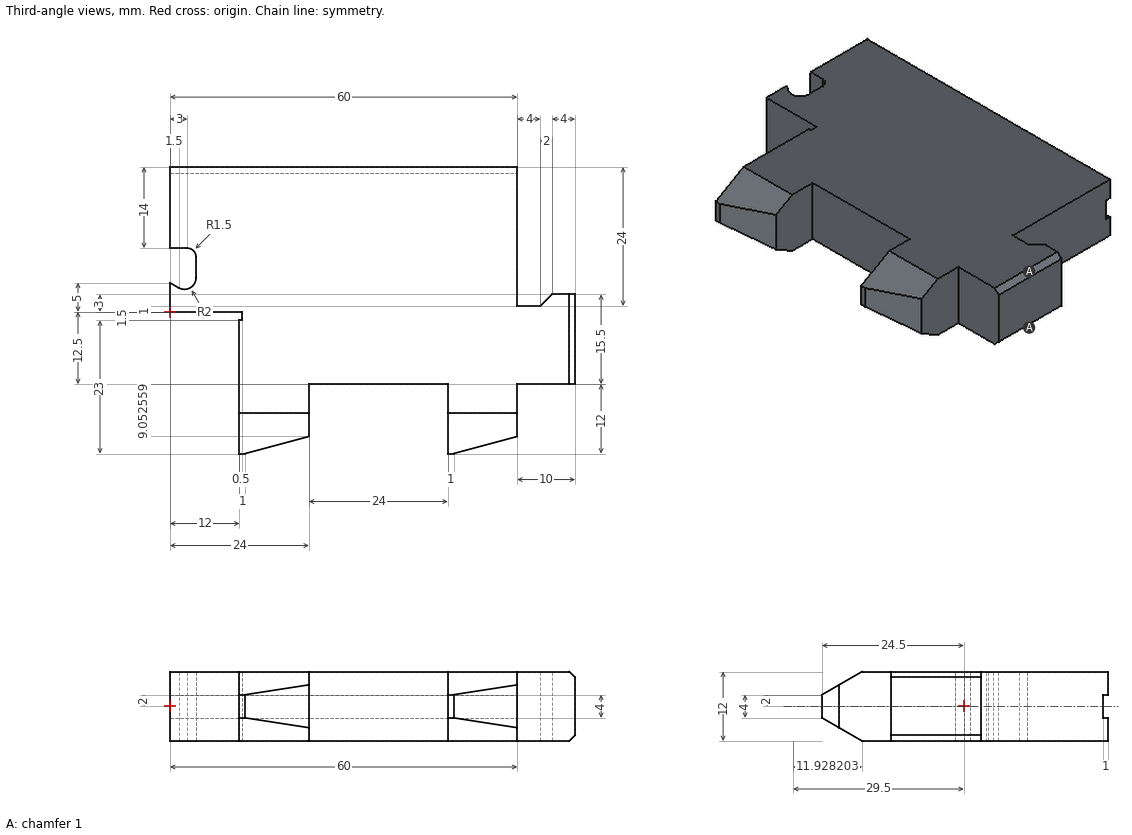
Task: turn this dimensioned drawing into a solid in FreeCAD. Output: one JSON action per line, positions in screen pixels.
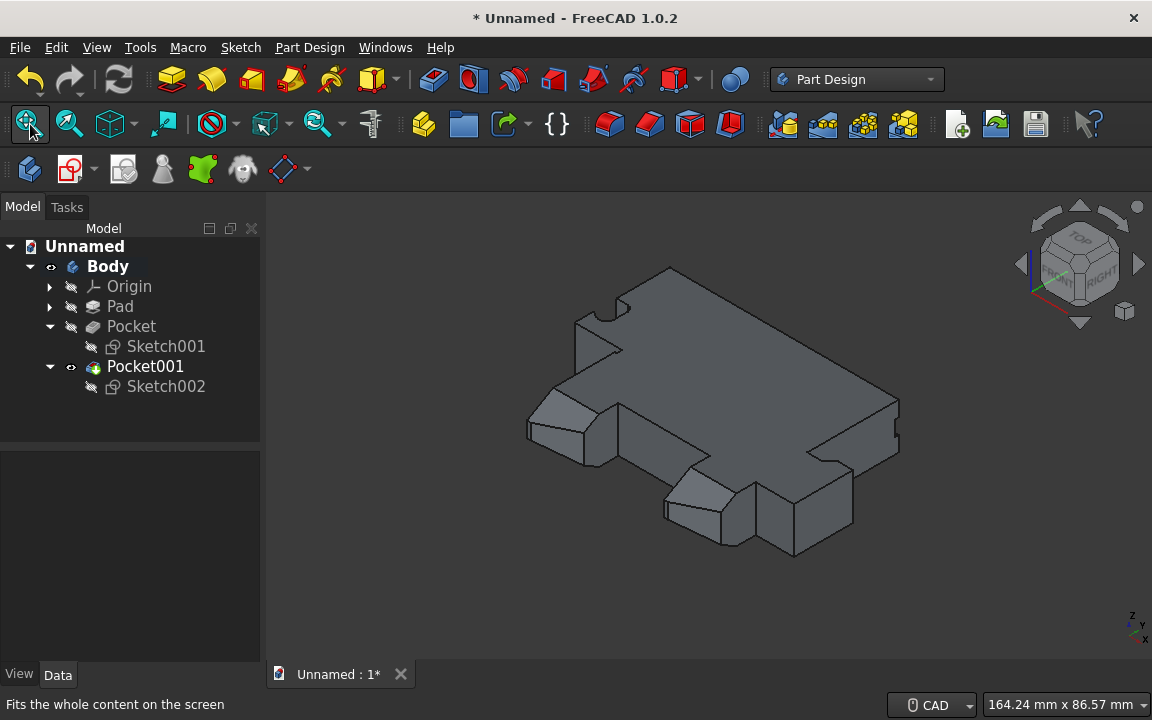
{"action": "left_click", "coordinate": [823, 486]}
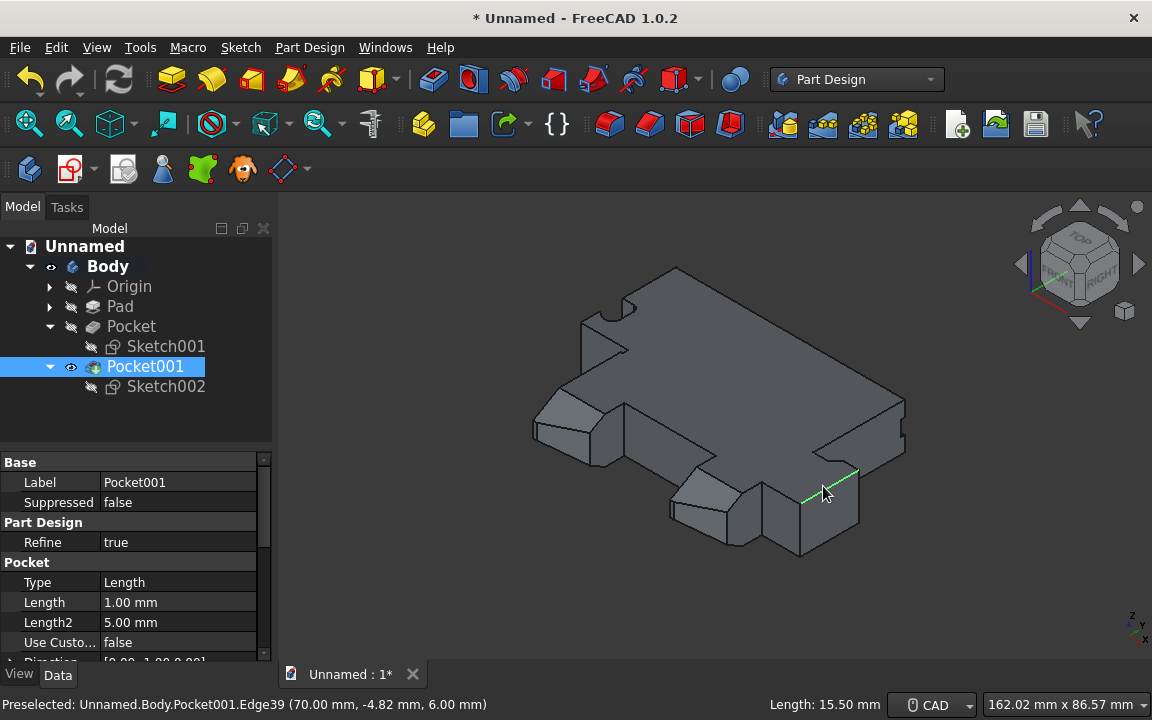
{"action": "key", "text": "2"}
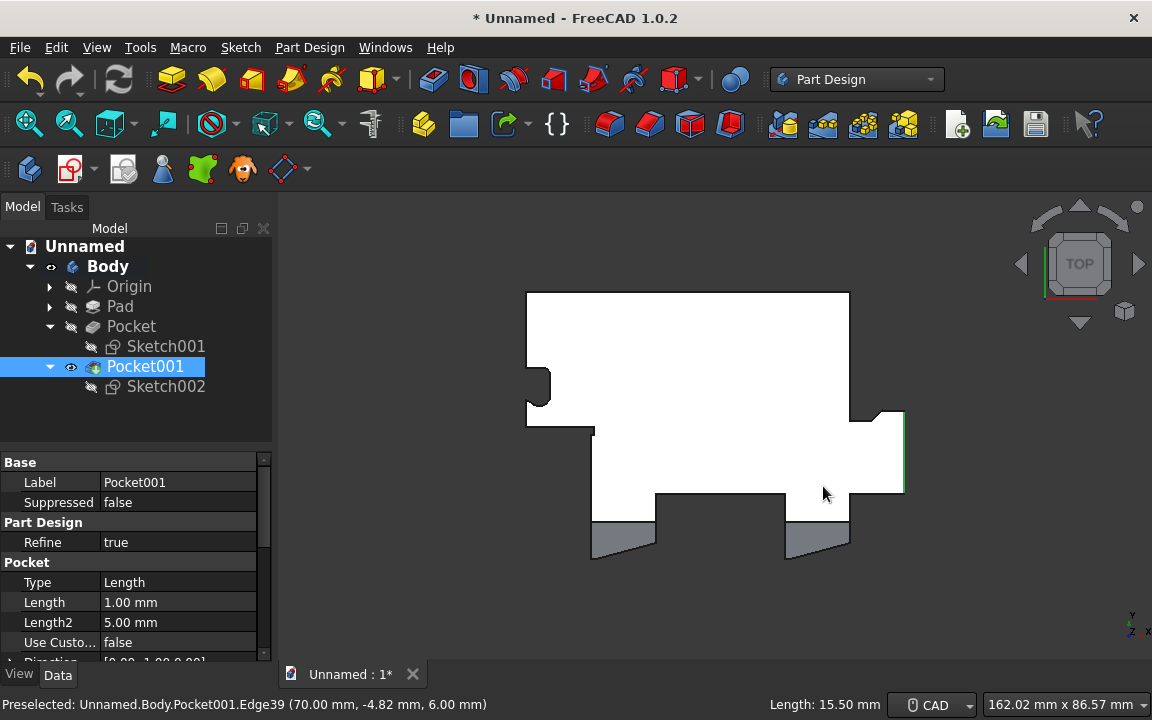
{"action": "key", "text": "1"}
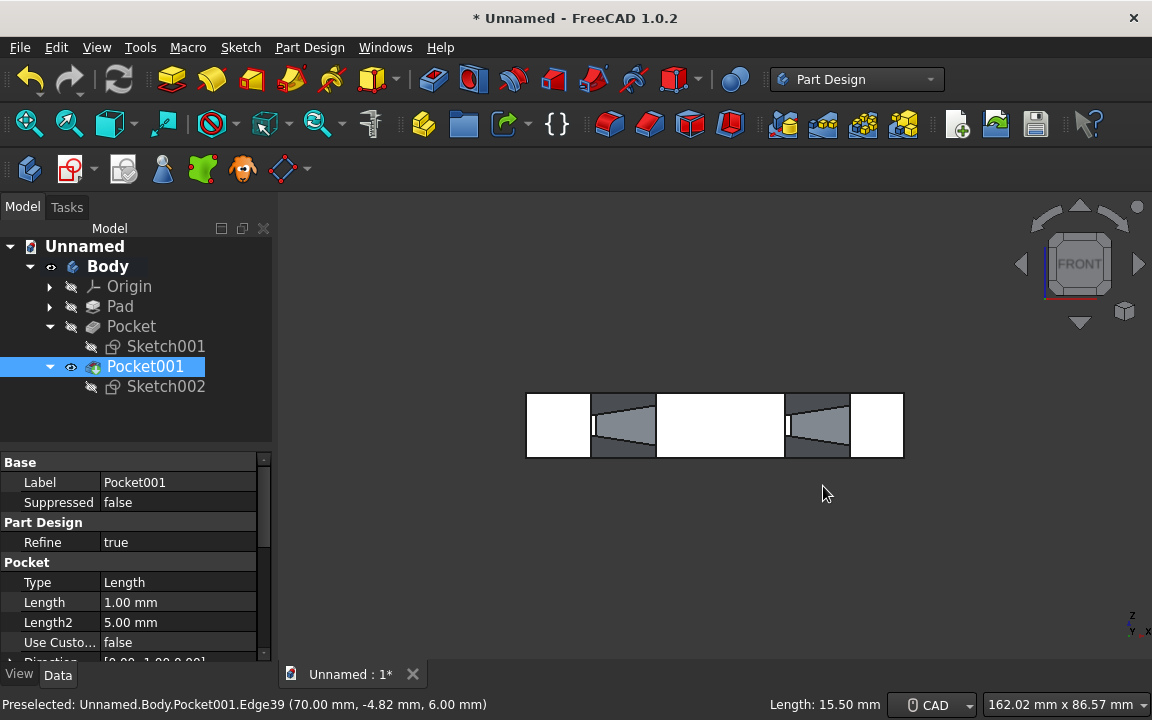
{"action": "left_click", "coordinate": [30, 124]}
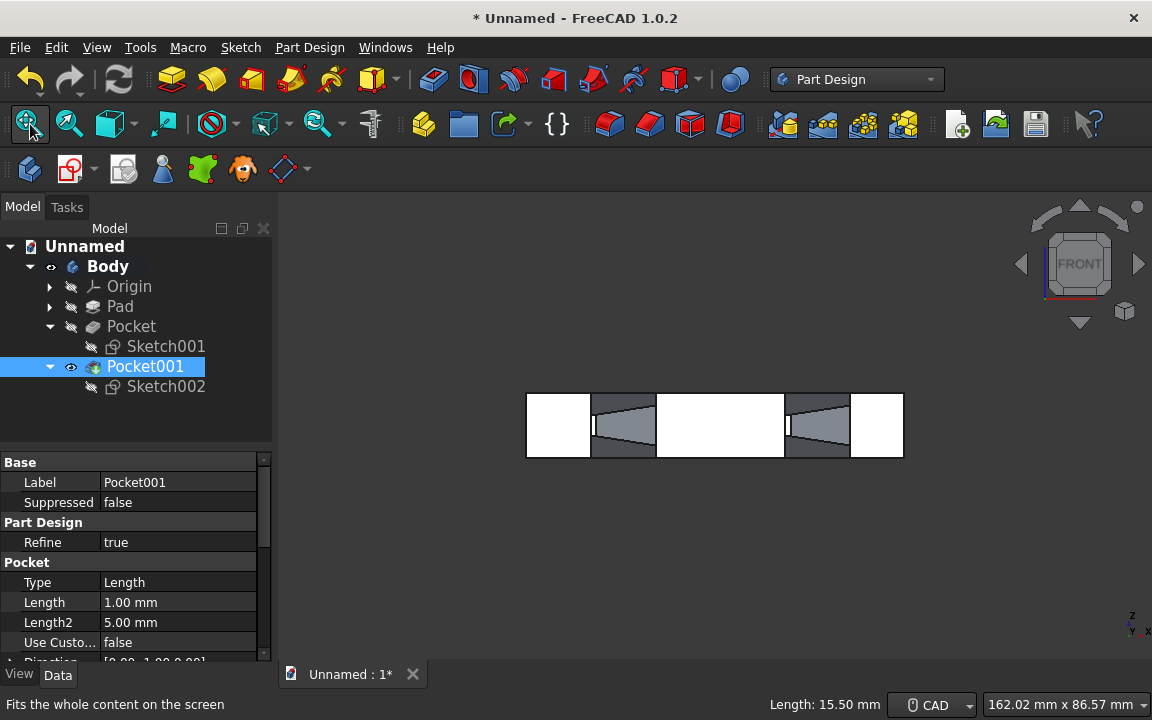
{"action": "key", "text": "3"}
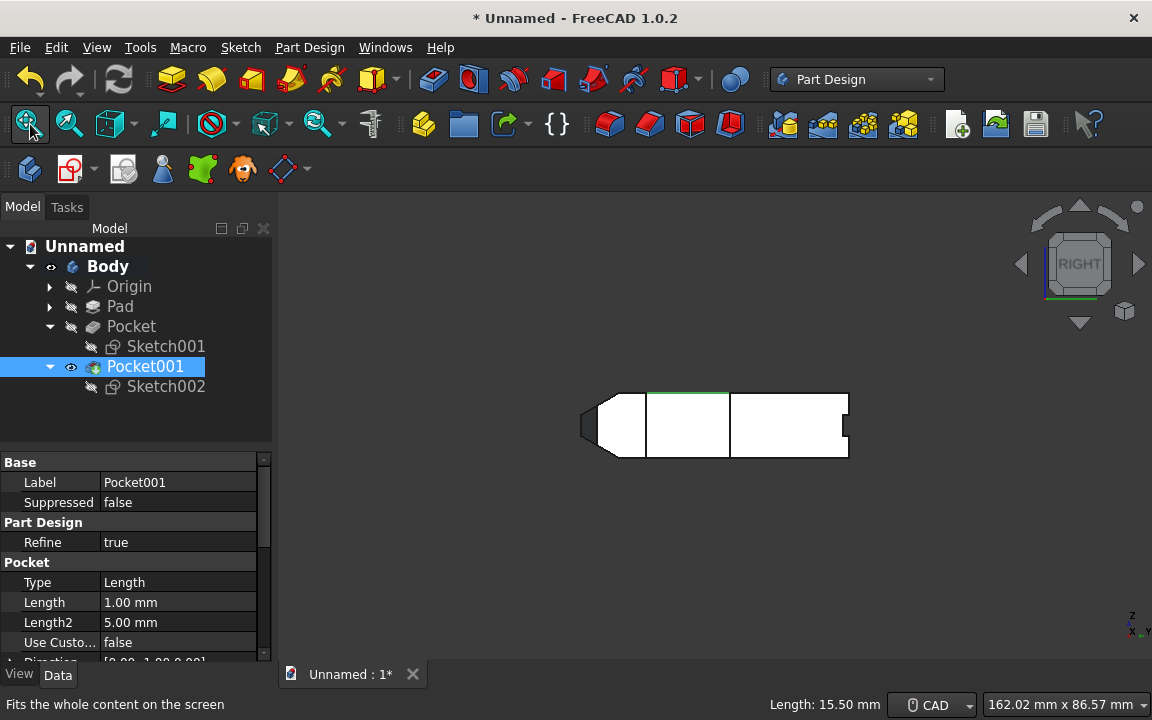
{"action": "left_click", "coordinate": [30, 124]}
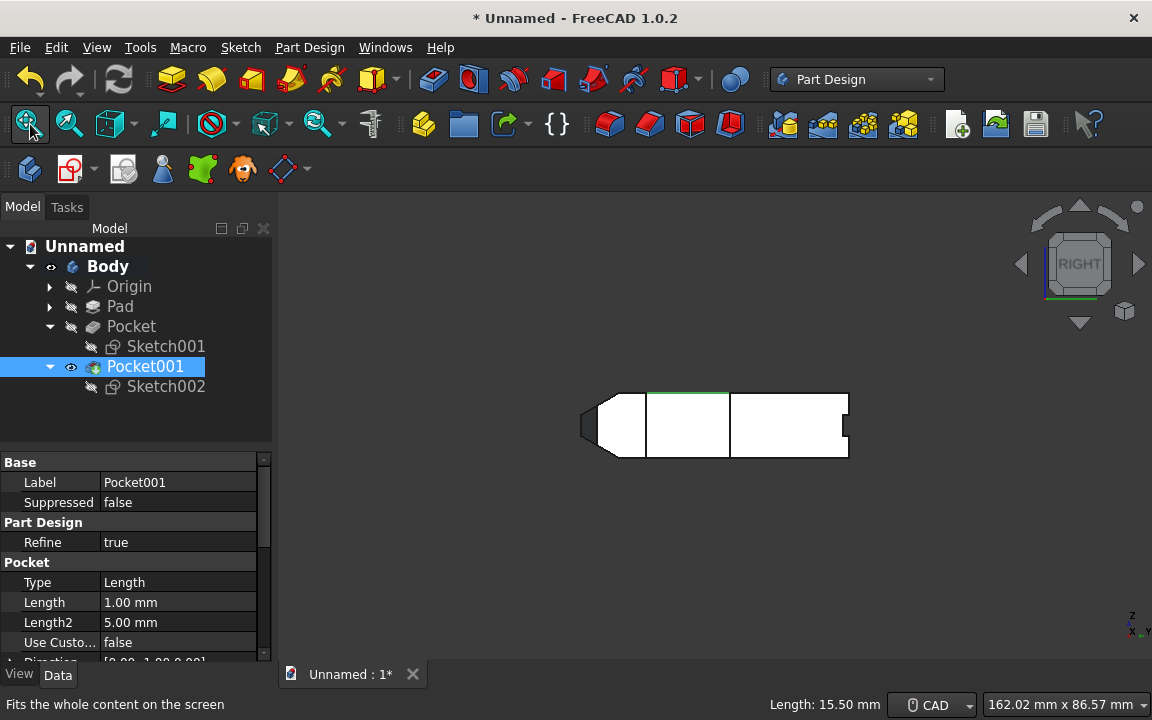
{"action": "left_click", "coordinate": [688, 457], "text": "ctrl"}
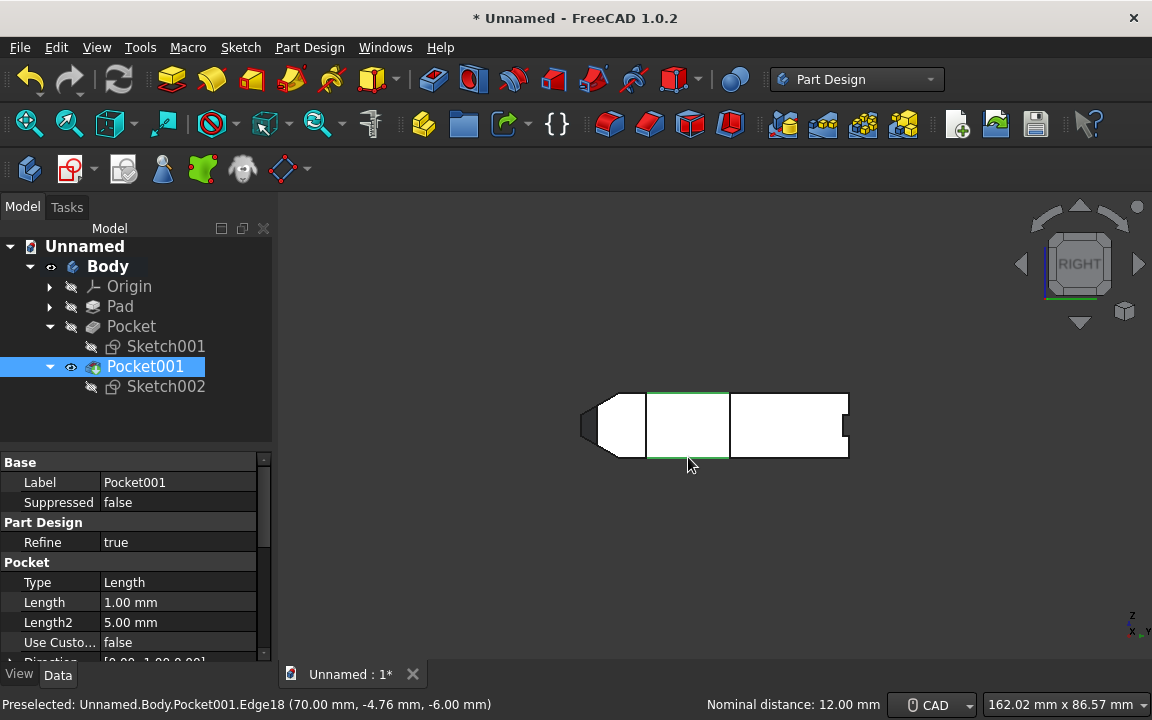
{"action": "left_click", "coordinate": [650, 124]}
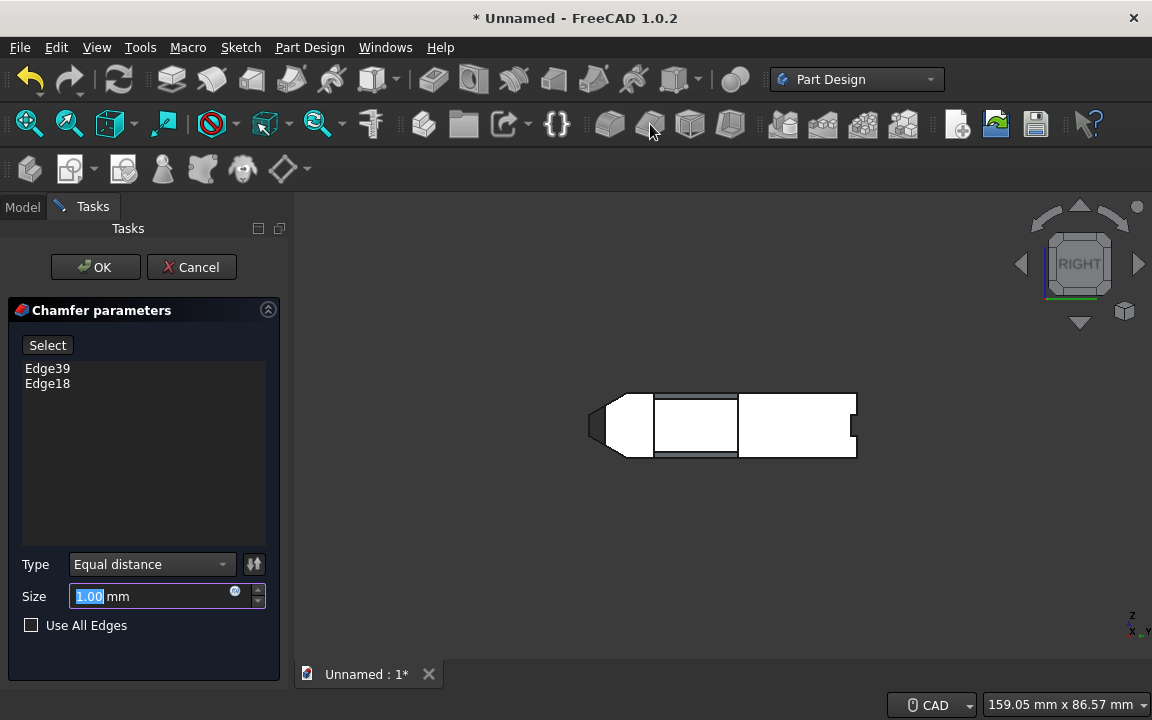
{"action": "type", "text": "1"}
{"action": "key", "text": "Tab"}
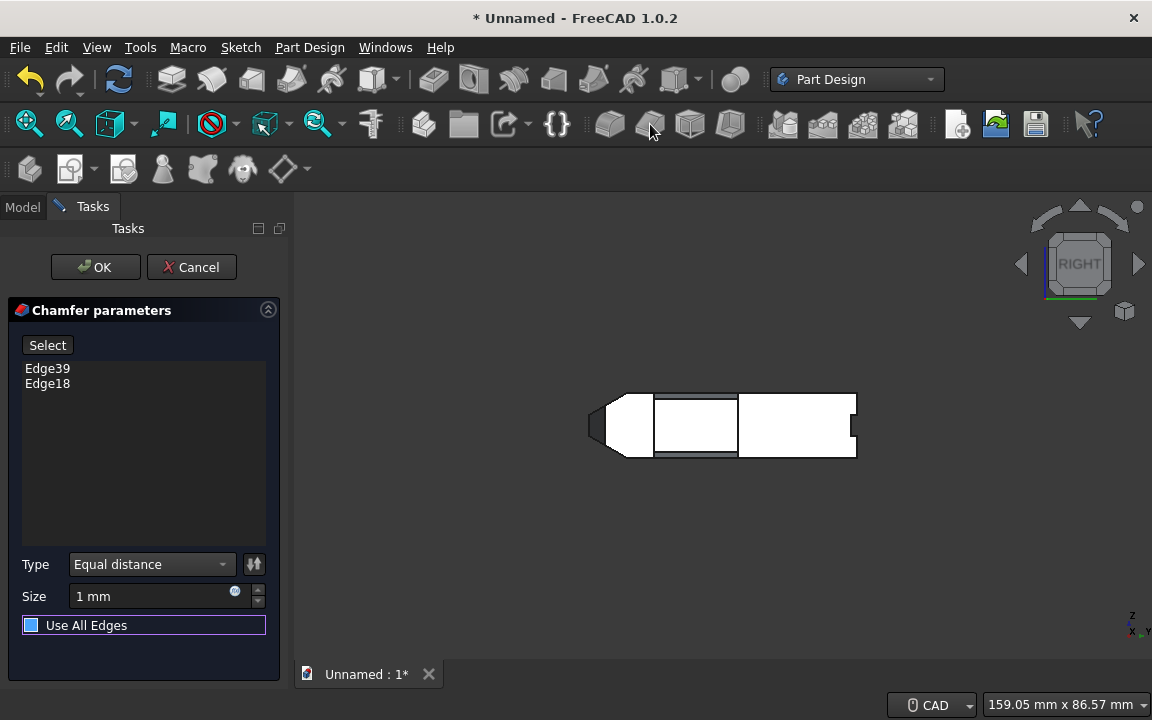
{"action": "left_click", "coordinate": [96, 267]}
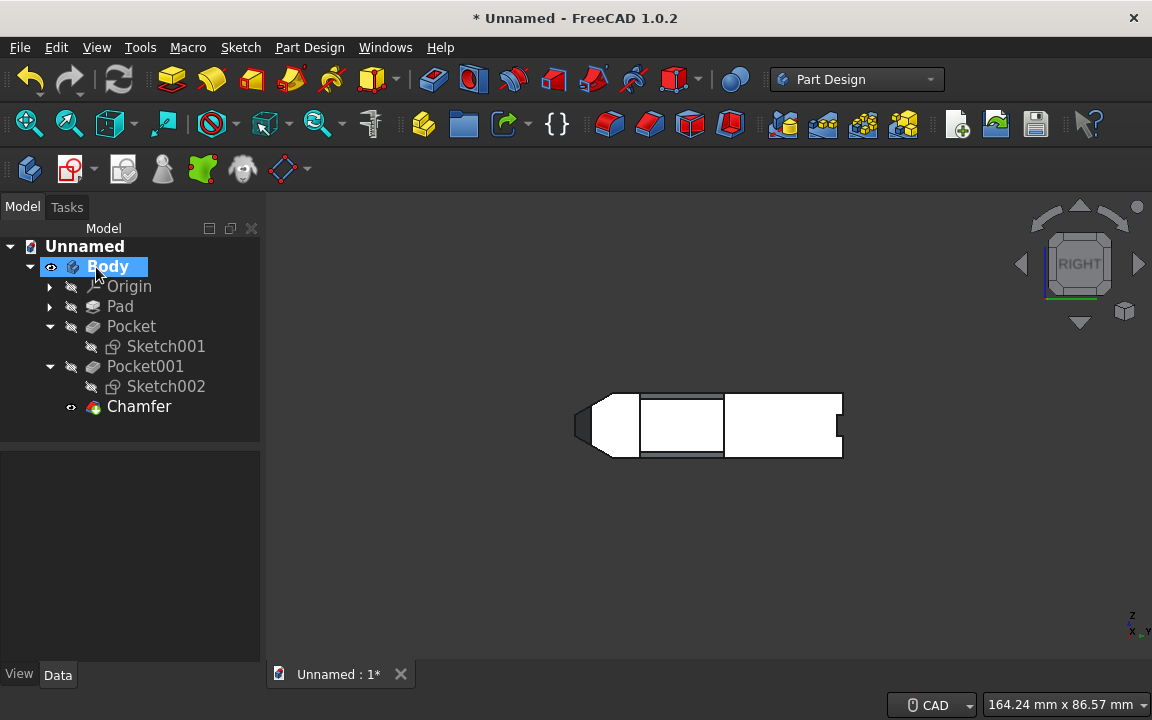
{"action": "key", "text": "0"}